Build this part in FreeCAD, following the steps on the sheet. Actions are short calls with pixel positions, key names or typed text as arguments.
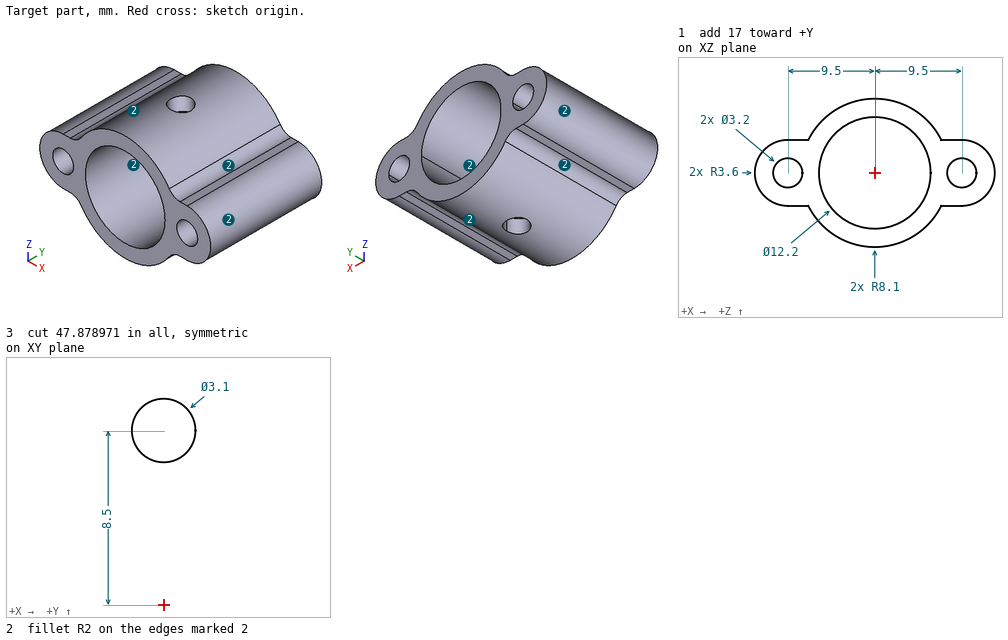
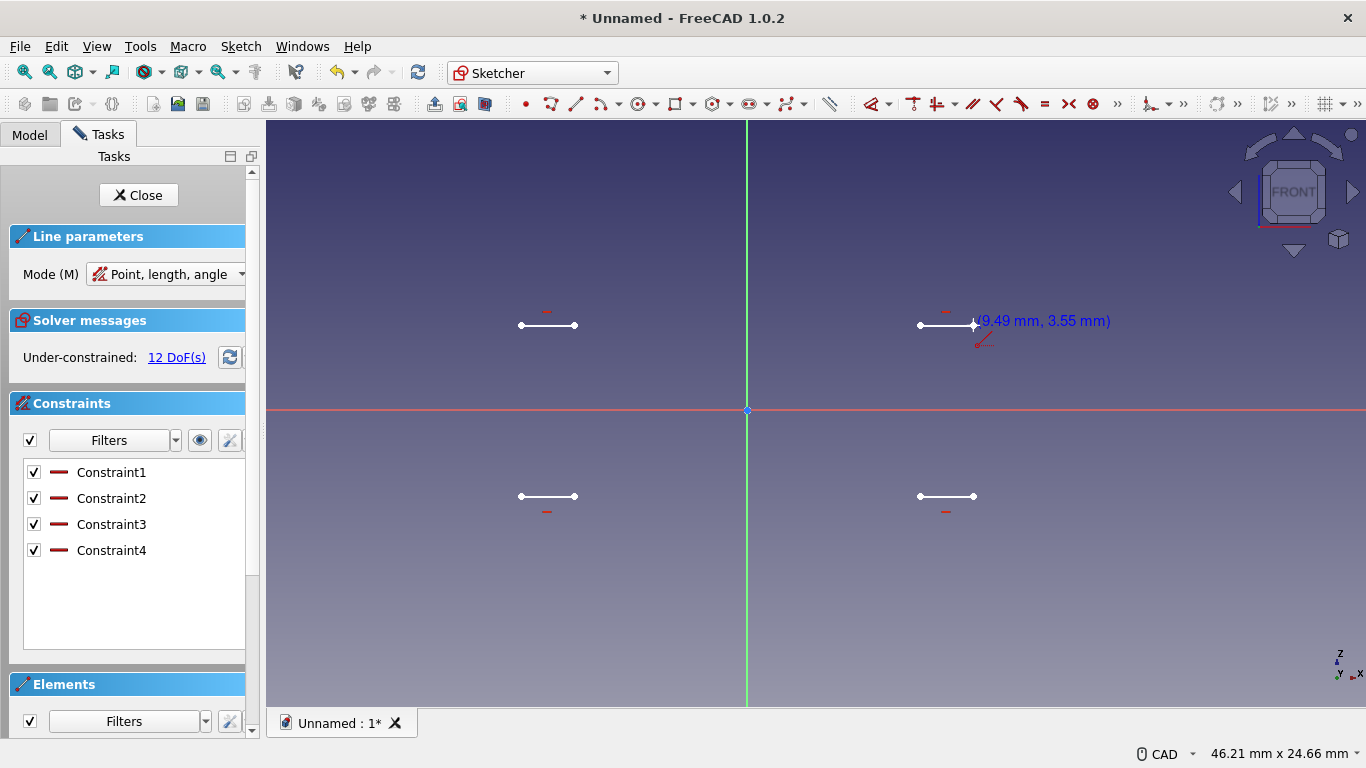
key(g)
key(3)
key(a)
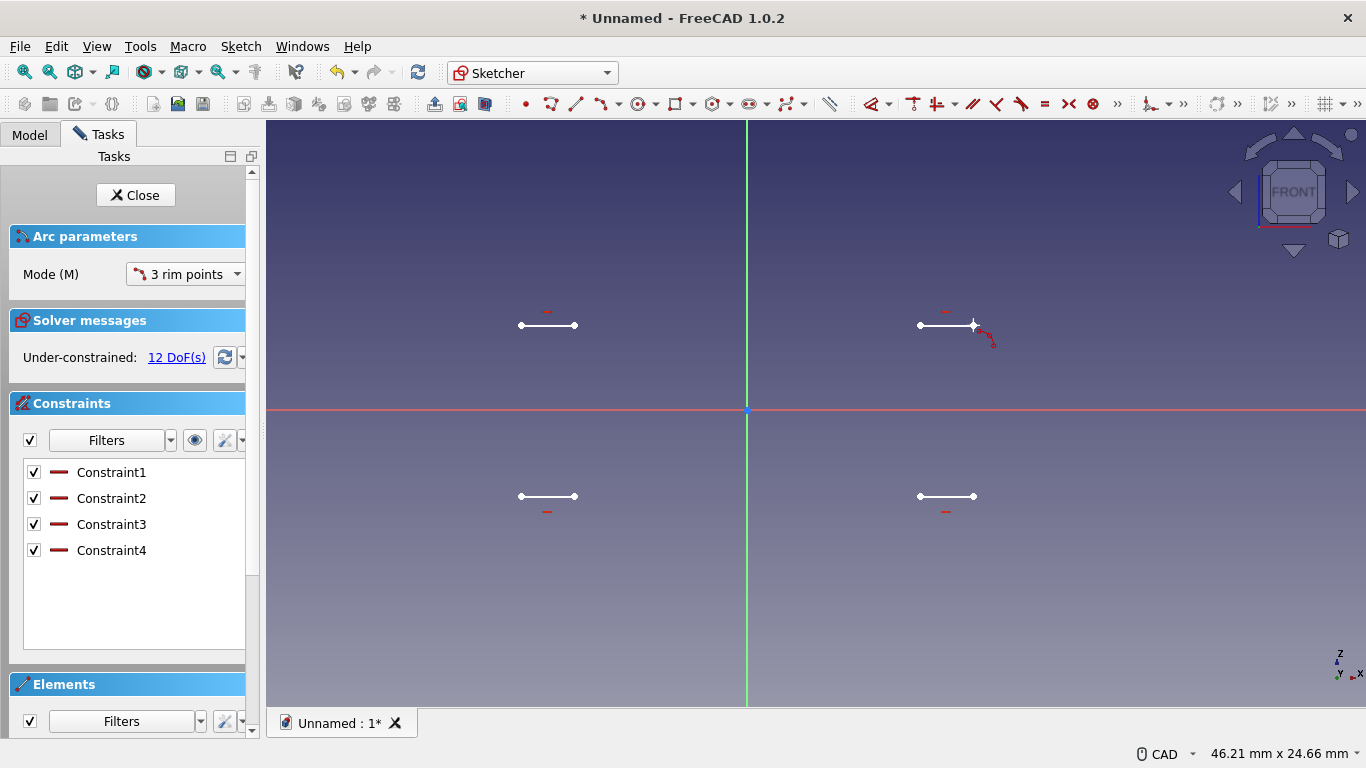
click(920, 497)
click(574, 497)
click(705, 599)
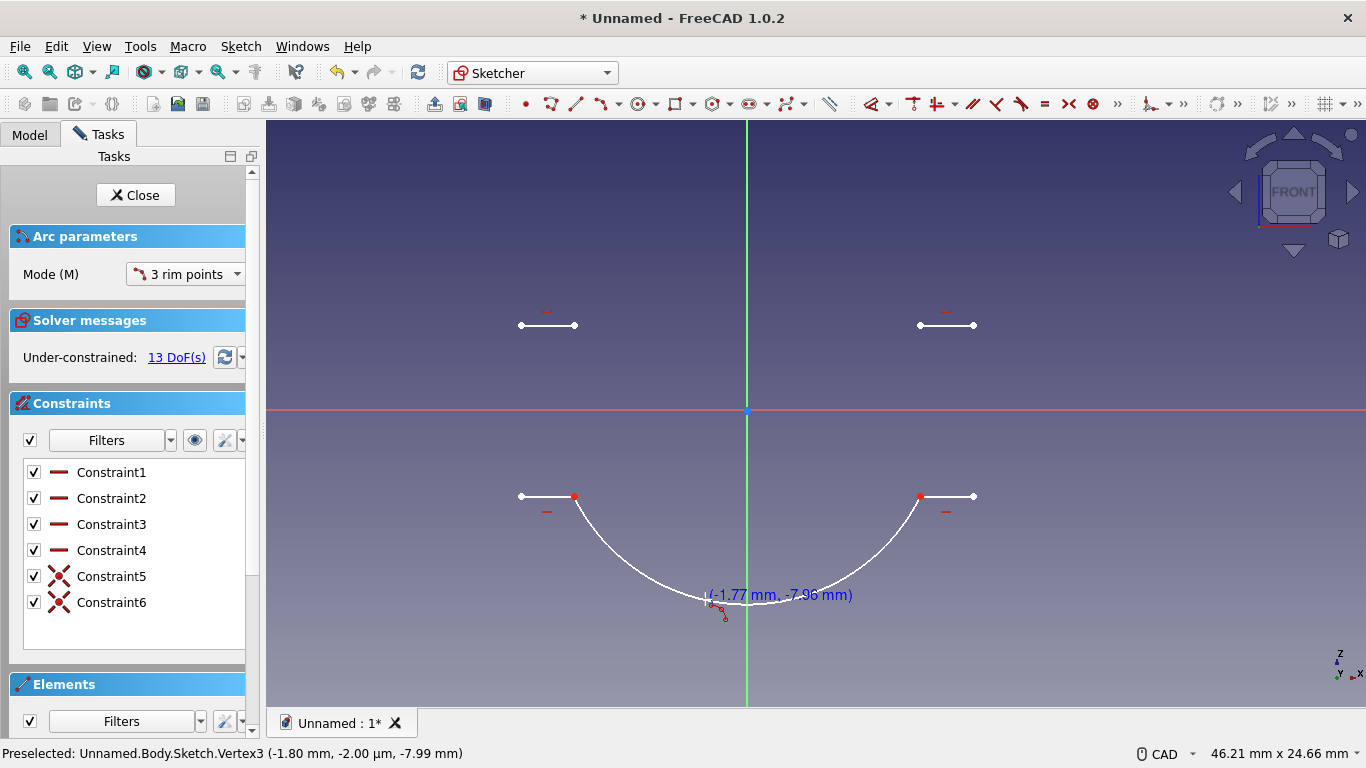
click(521, 497)
click(521, 326)
click(440, 384)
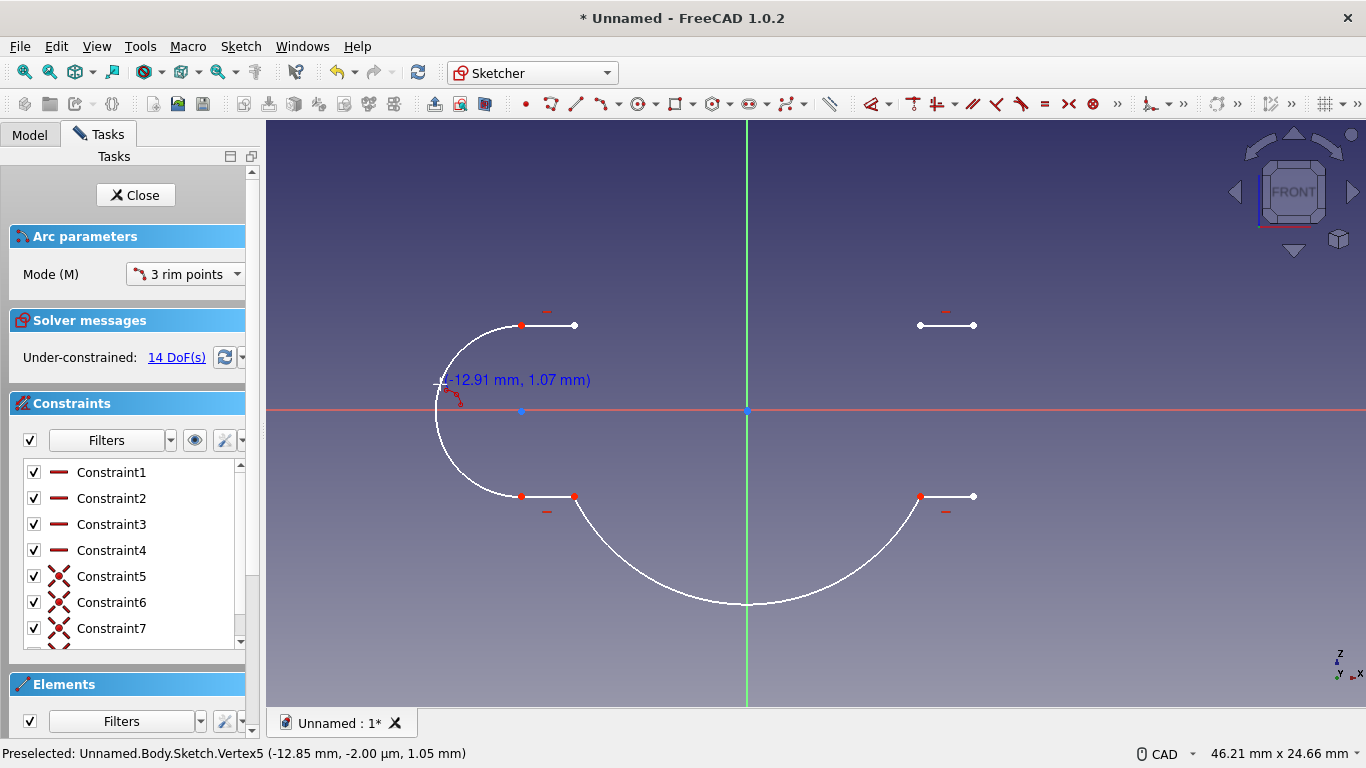
click(574, 326)
click(920, 326)
click(790, 222)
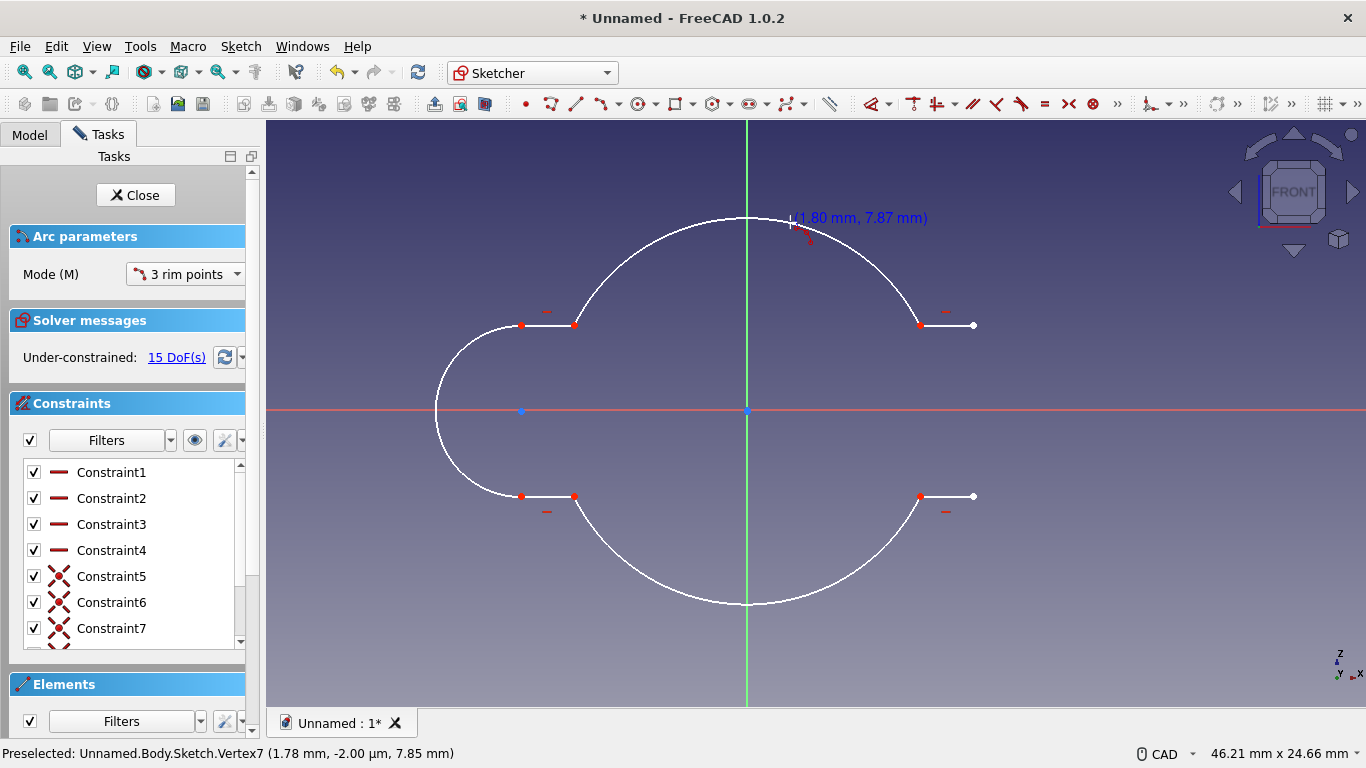
click(973, 326)
click(973, 497)
click(1055, 437)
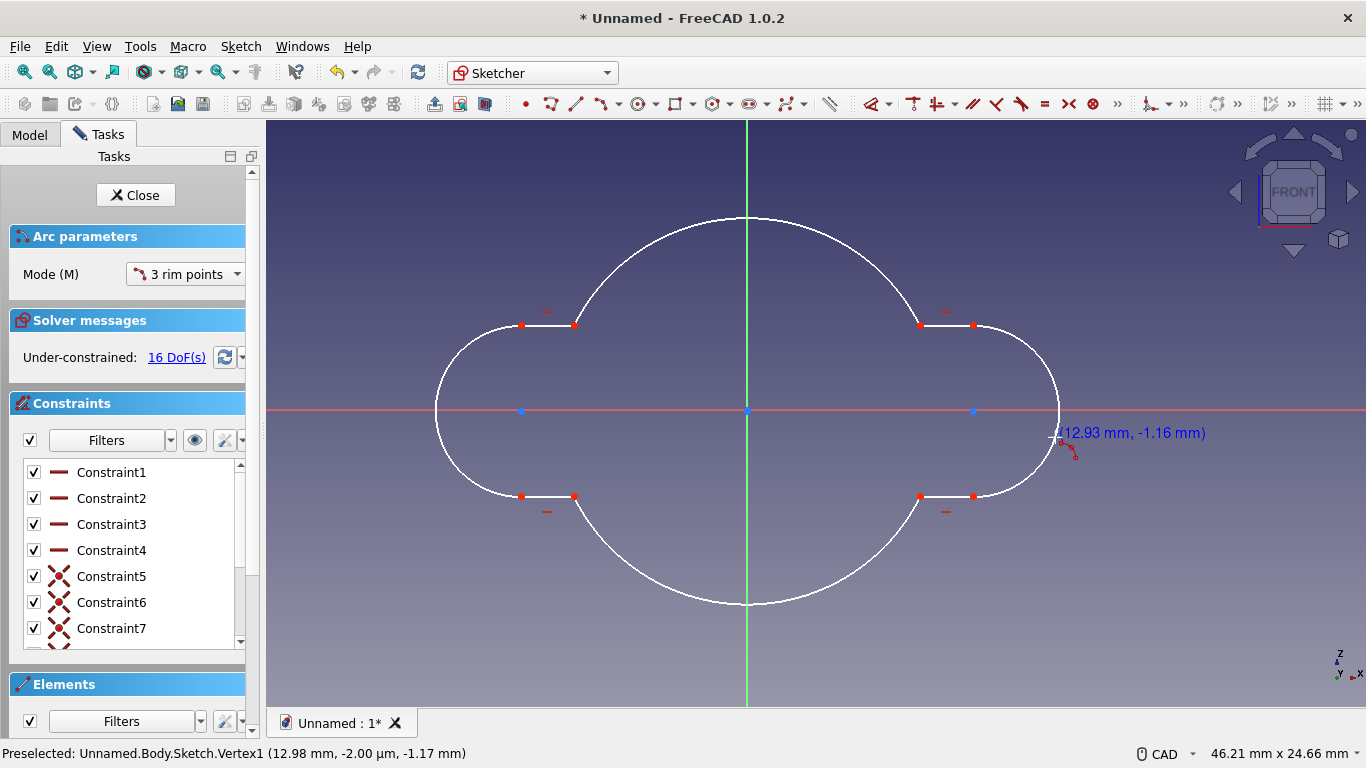
click(638, 104)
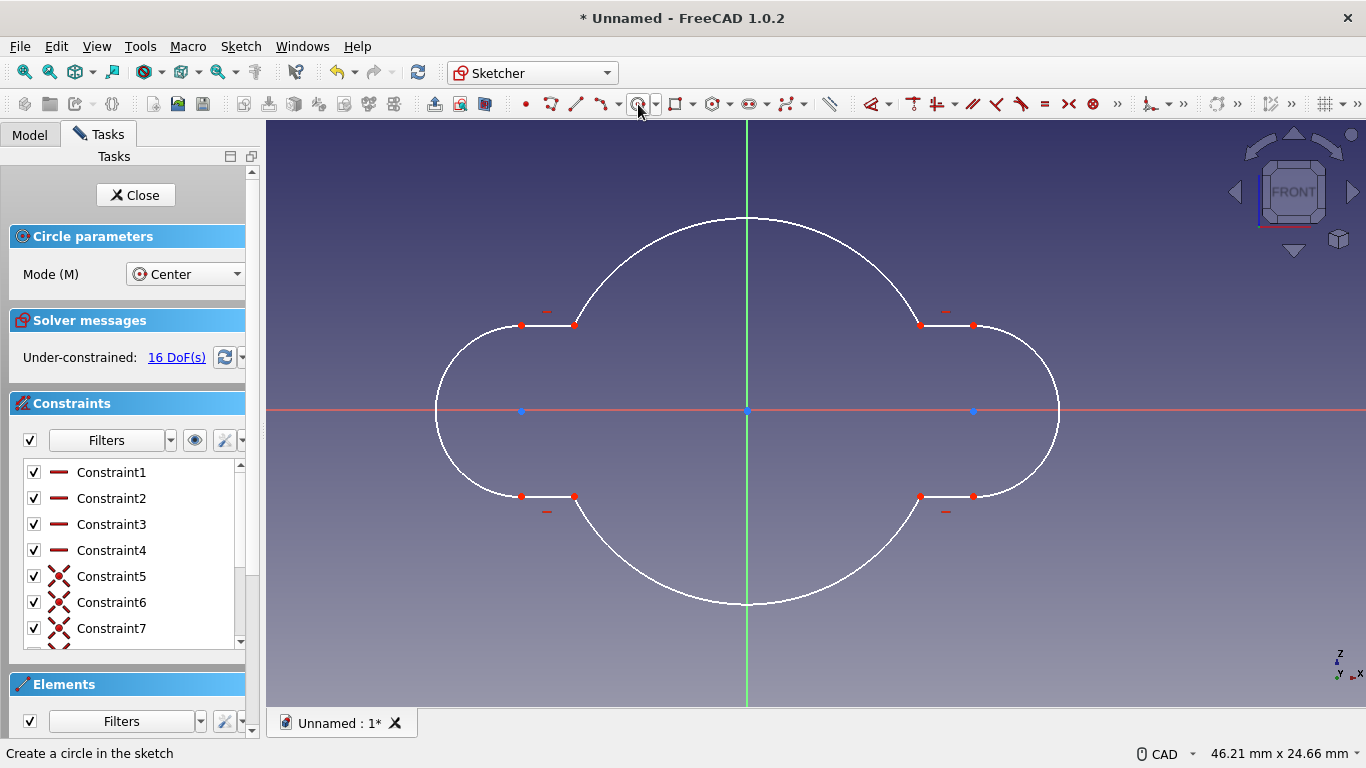
click(521, 410)
click(548, 384)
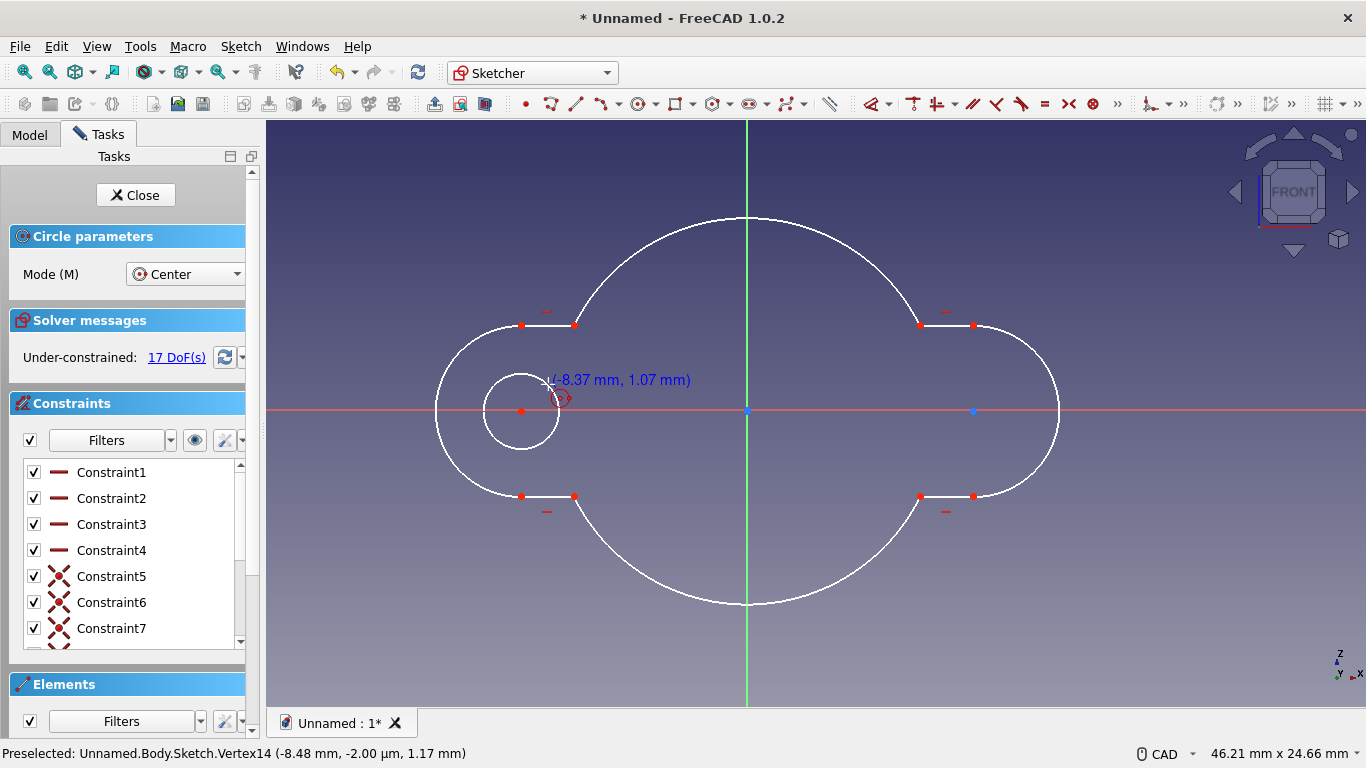
click(747, 410)
click(850, 308)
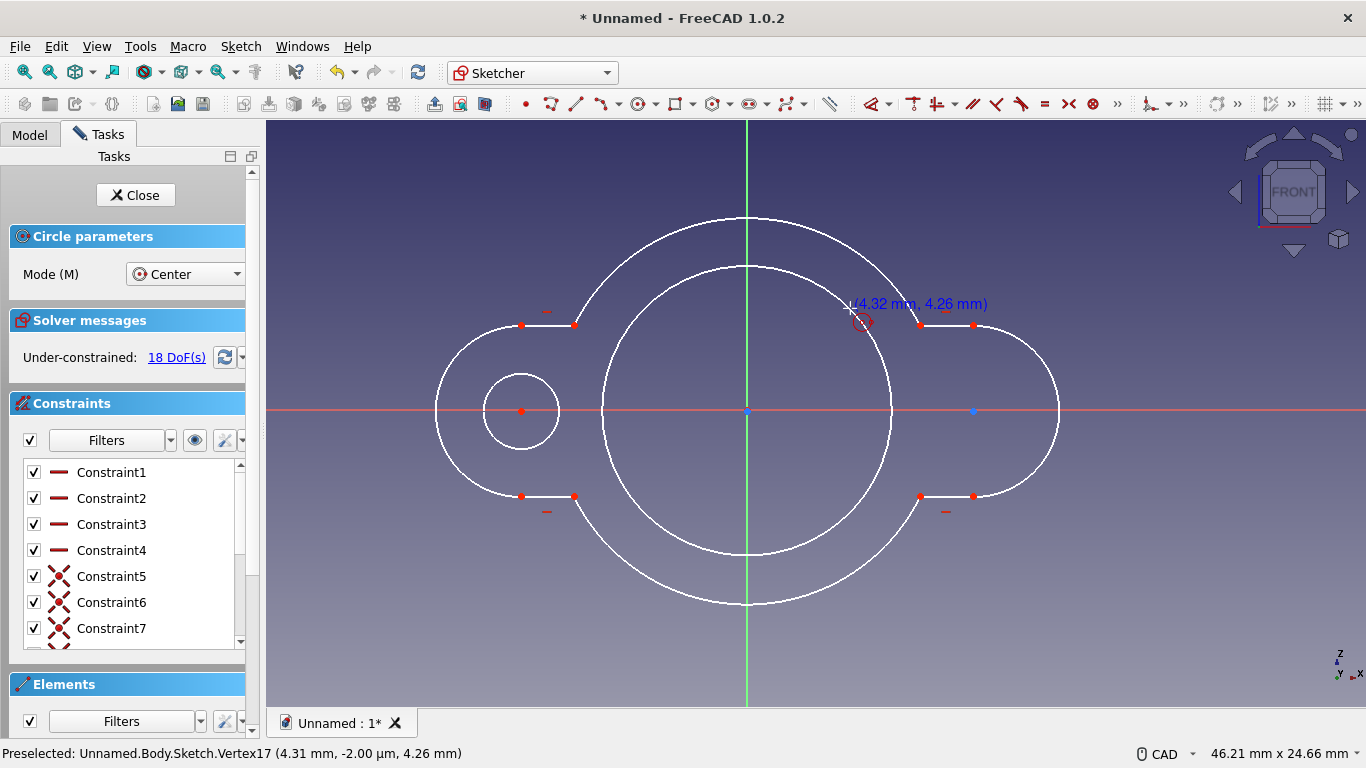
click(973, 410)
click(1000, 384)
key(Escape)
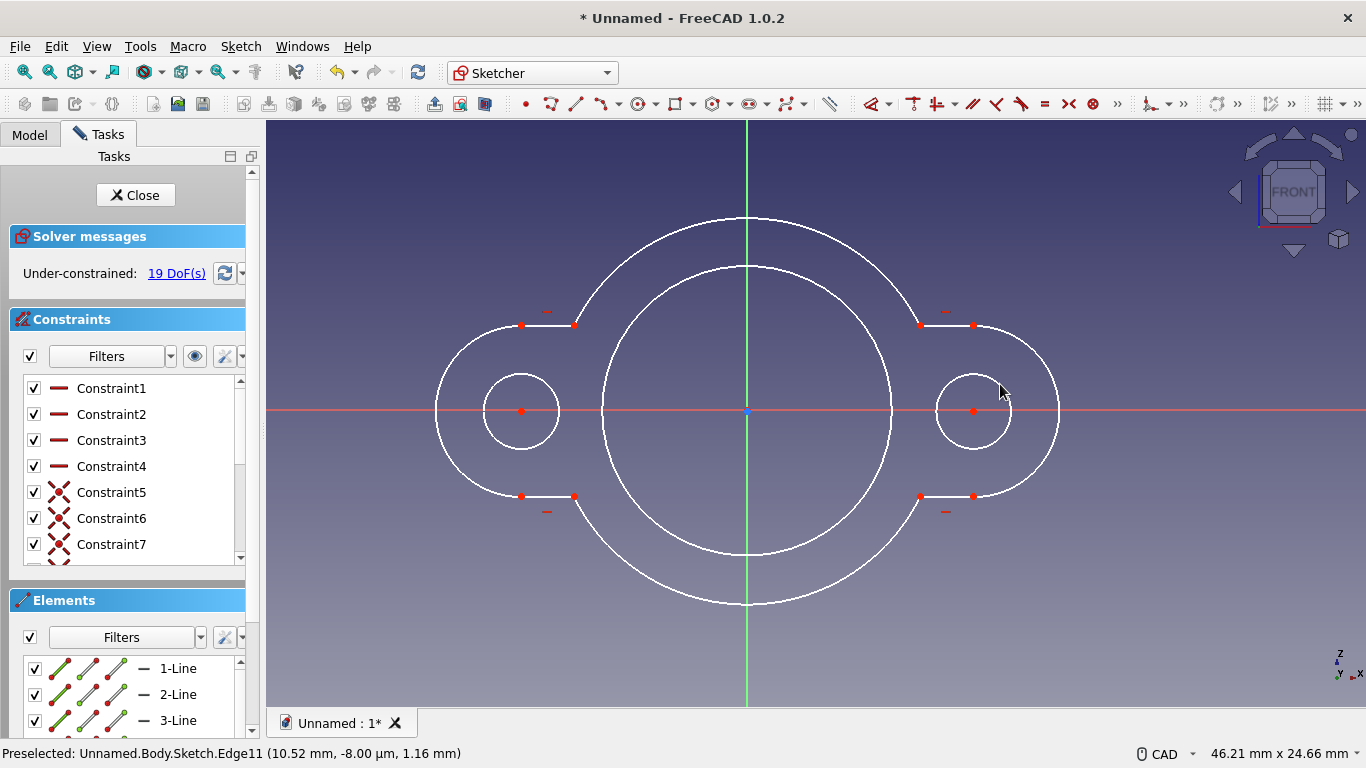
click(957, 497)